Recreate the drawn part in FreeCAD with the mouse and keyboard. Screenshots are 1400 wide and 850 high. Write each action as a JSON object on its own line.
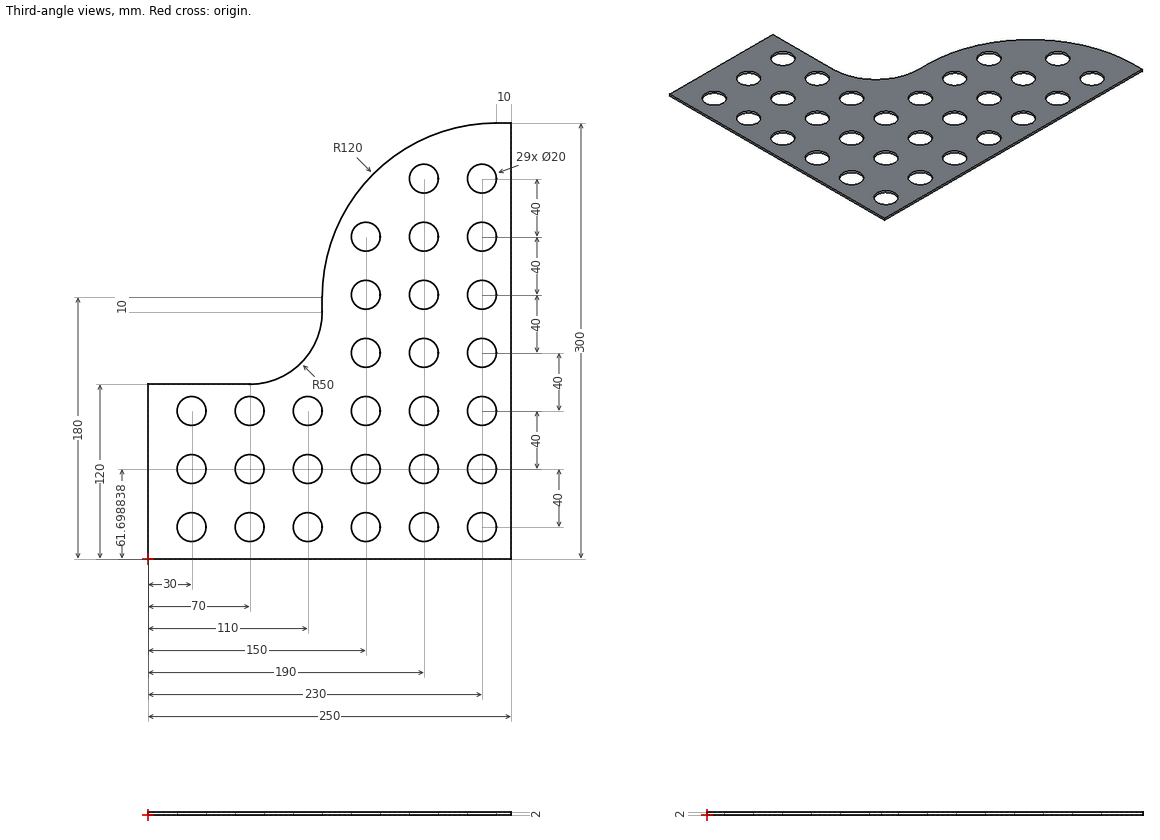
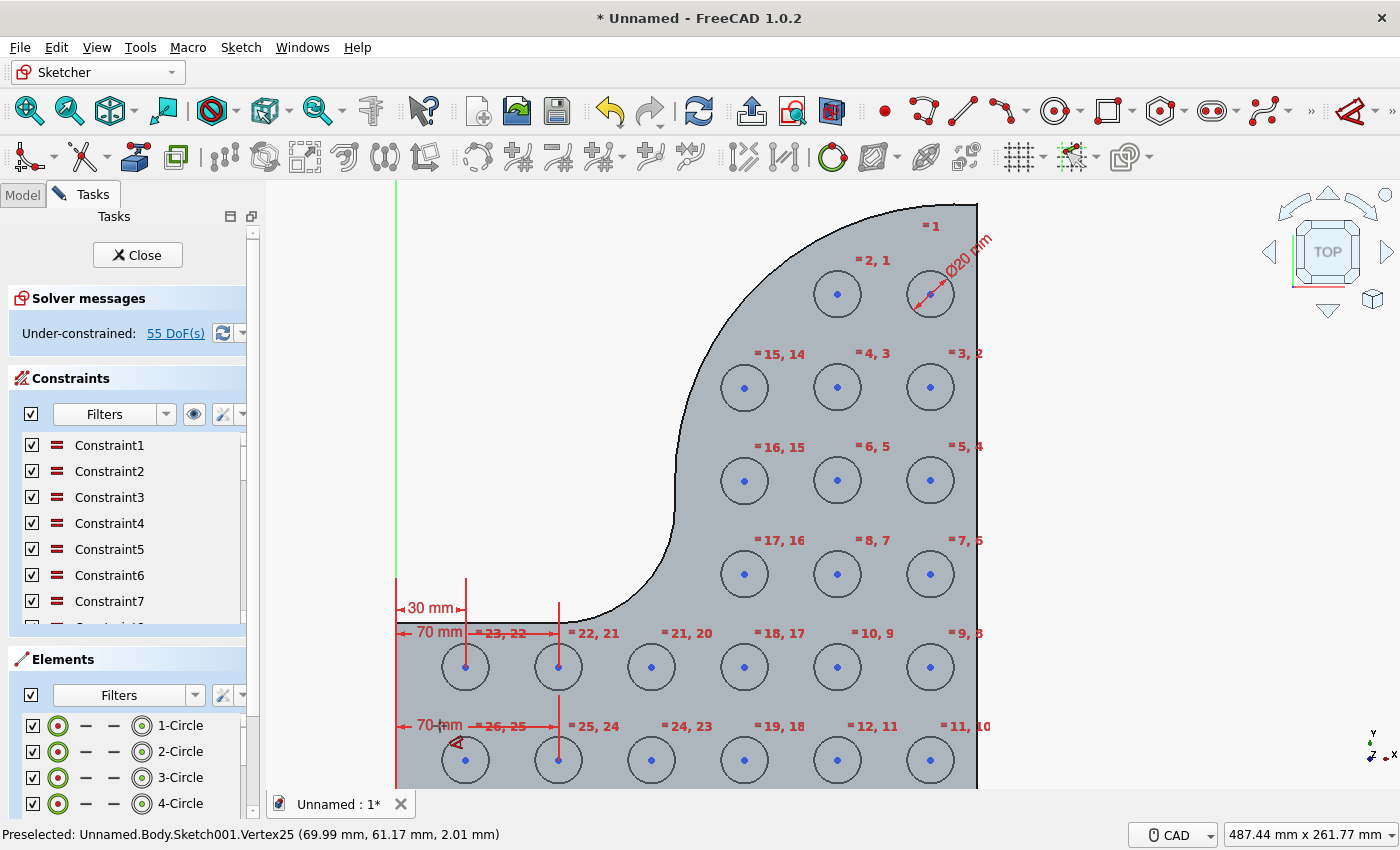
{"action": "left_click", "coordinate": [466, 760]}
{"action": "left_click", "coordinate": [431, 702]}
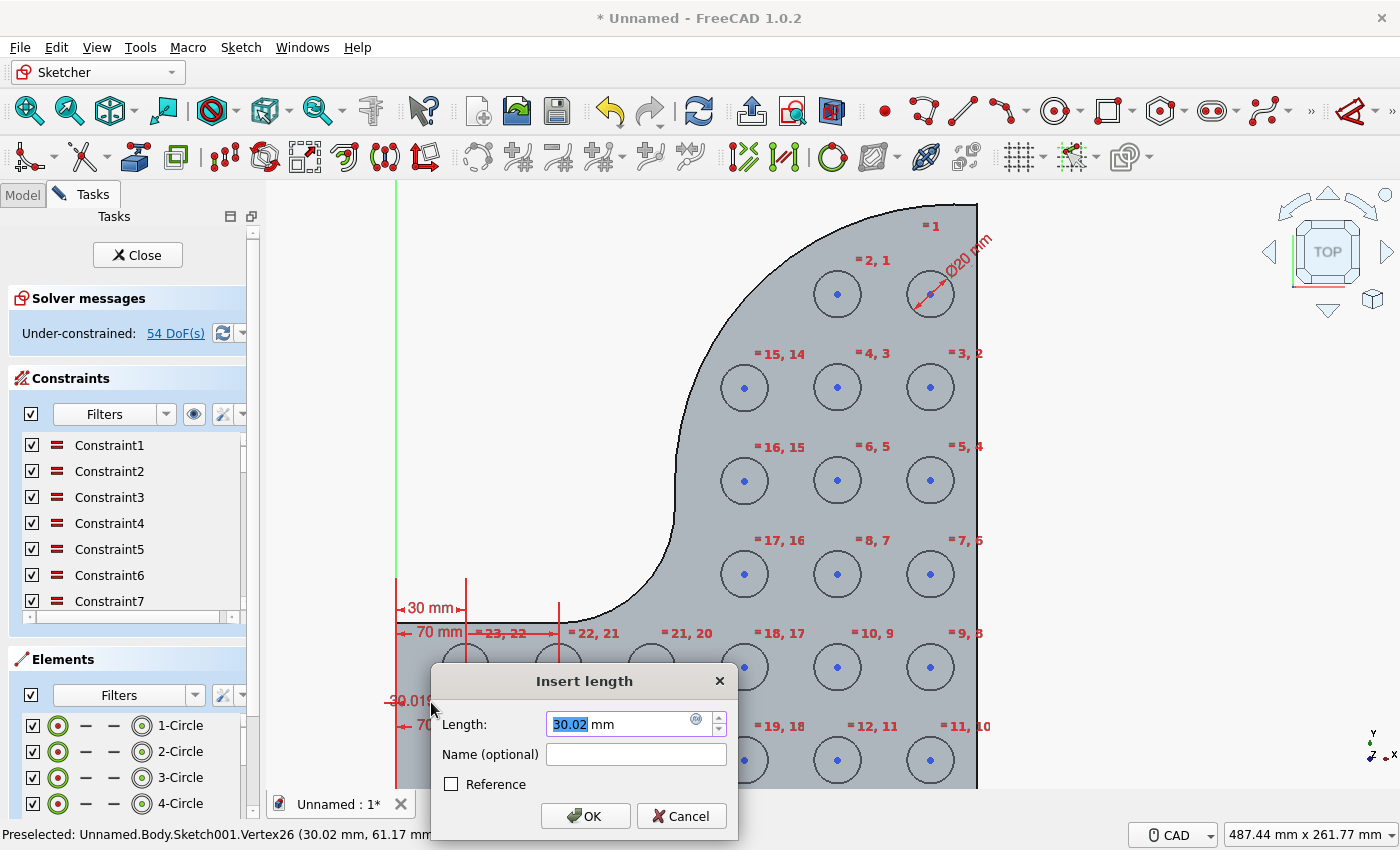
{"action": "type", "text": "30"}
{"action": "key", "text": "Return"}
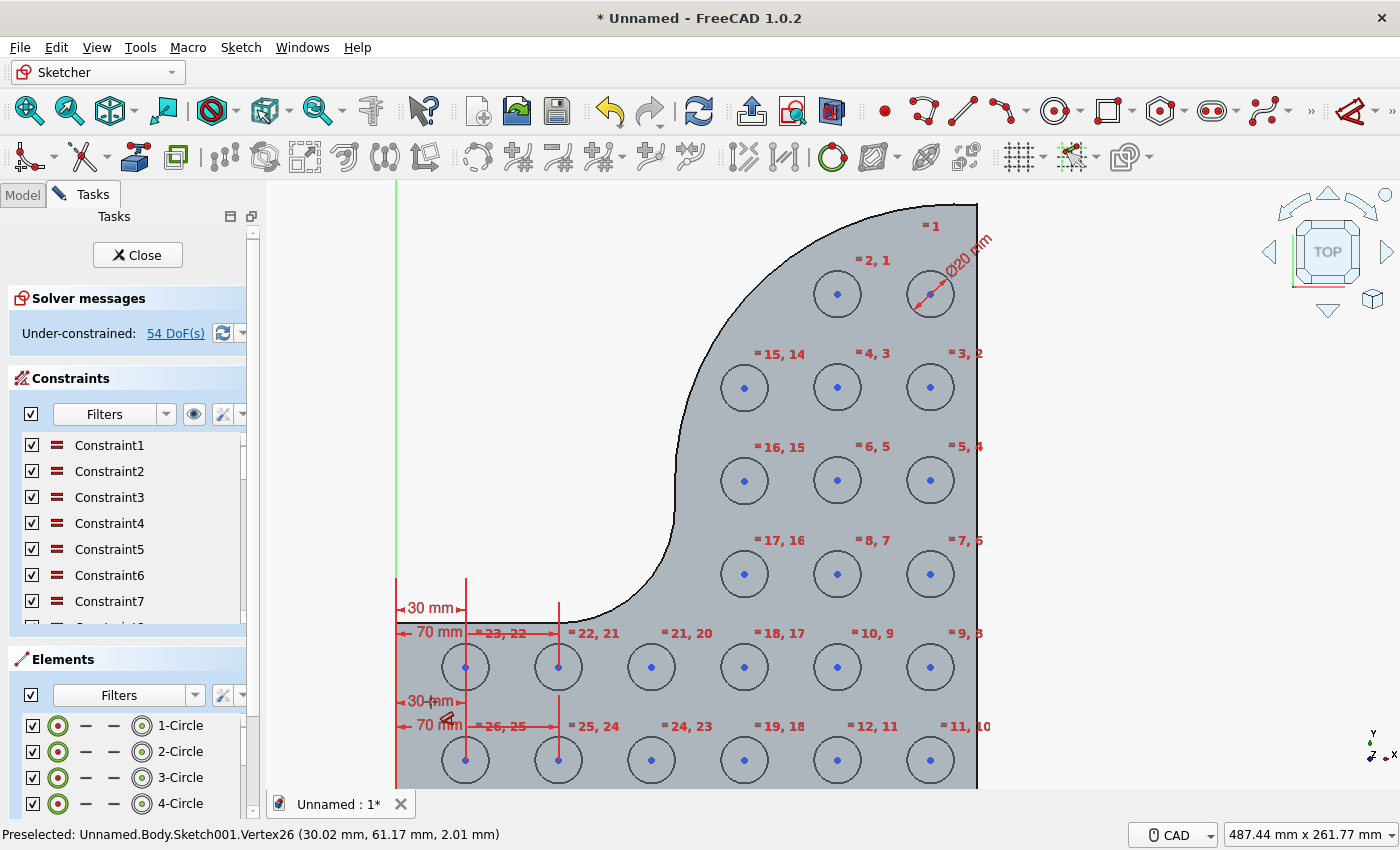
{"action": "scroll", "coordinate": [947, 277], "scroll_direction": "down", "scroll_amount": 2}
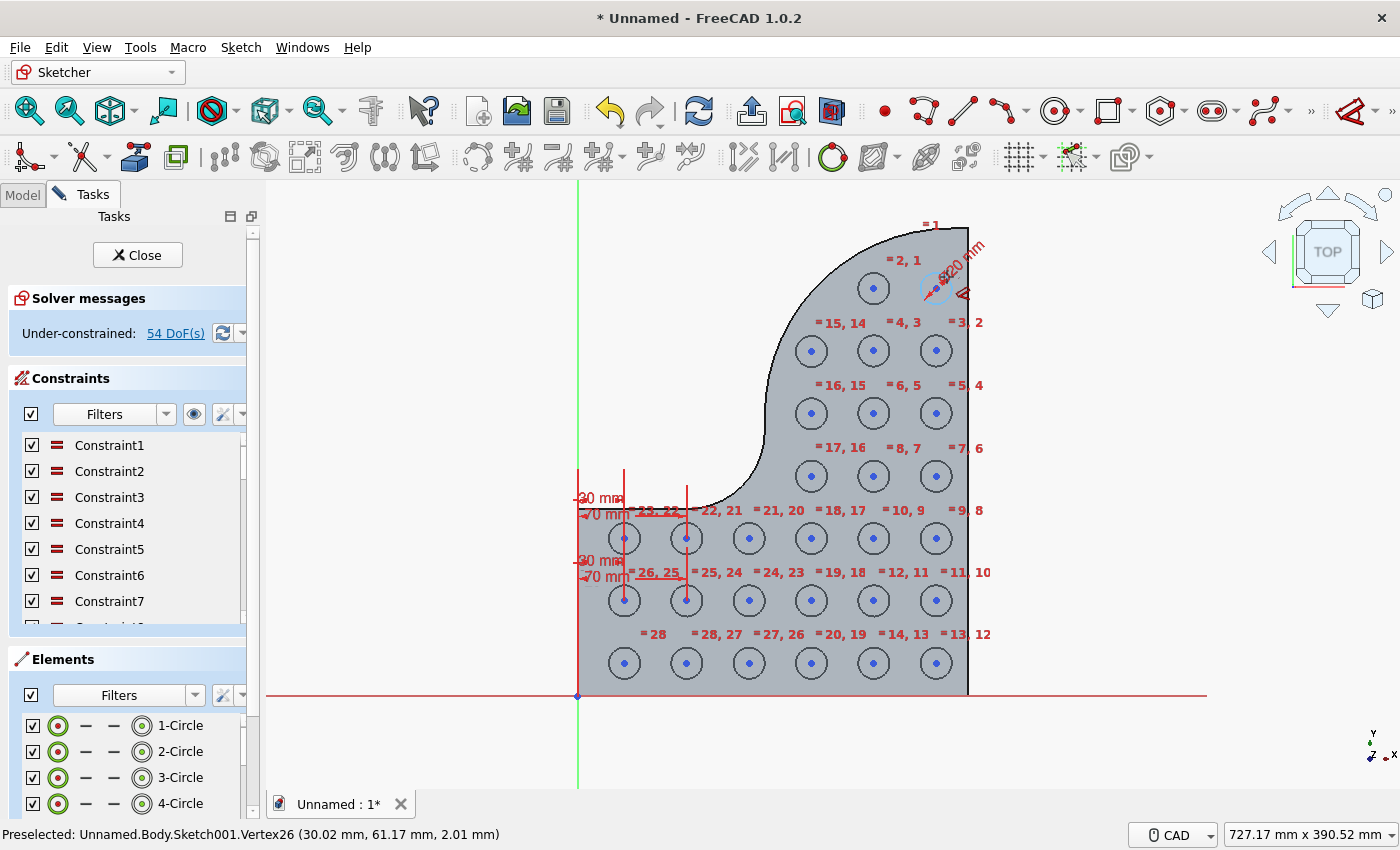
{"action": "left_click", "coordinate": [687, 663]}
{"action": "left_click", "coordinate": [632, 730]}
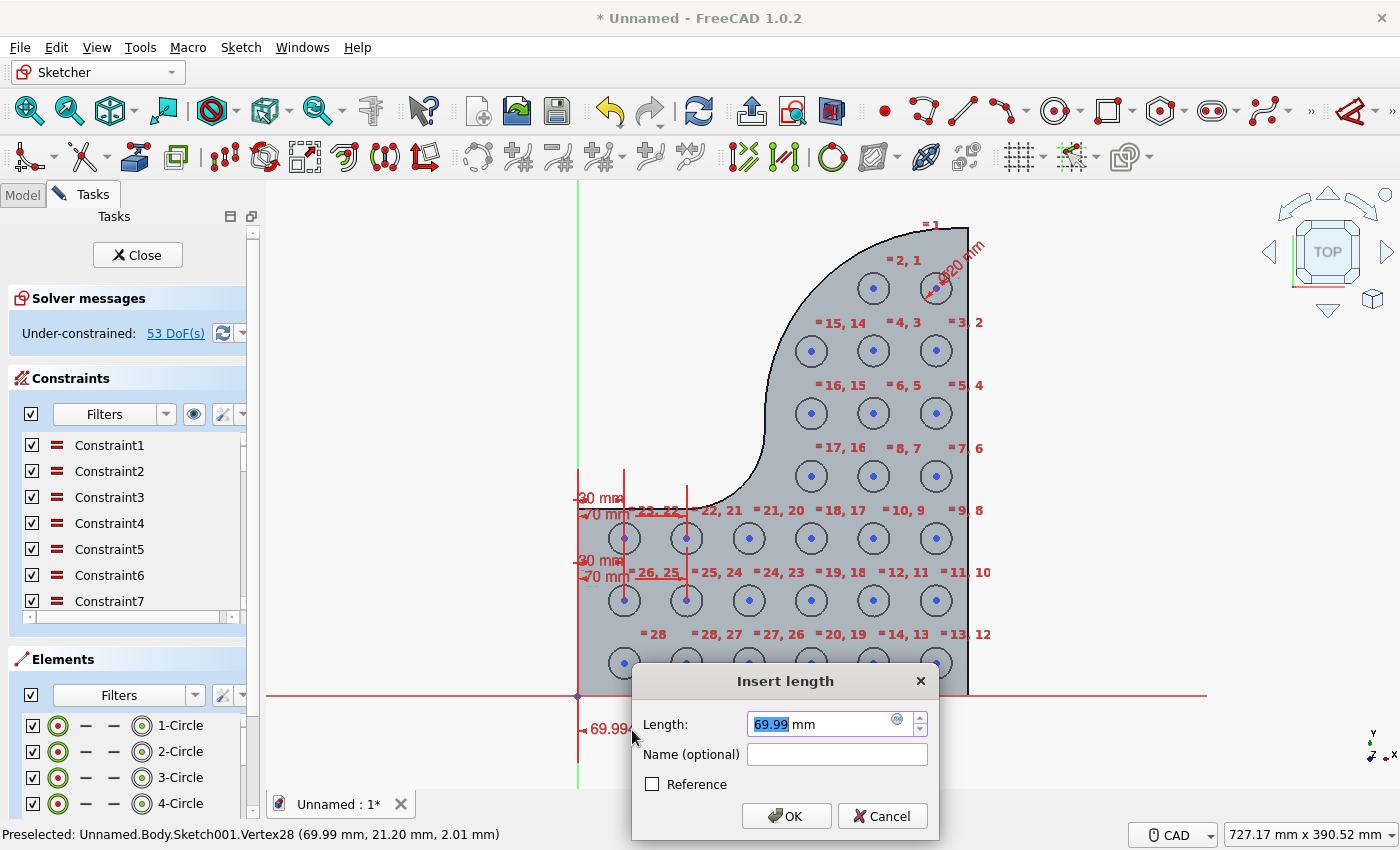
{"action": "type", "text": "70"}
{"action": "key", "text": "Return"}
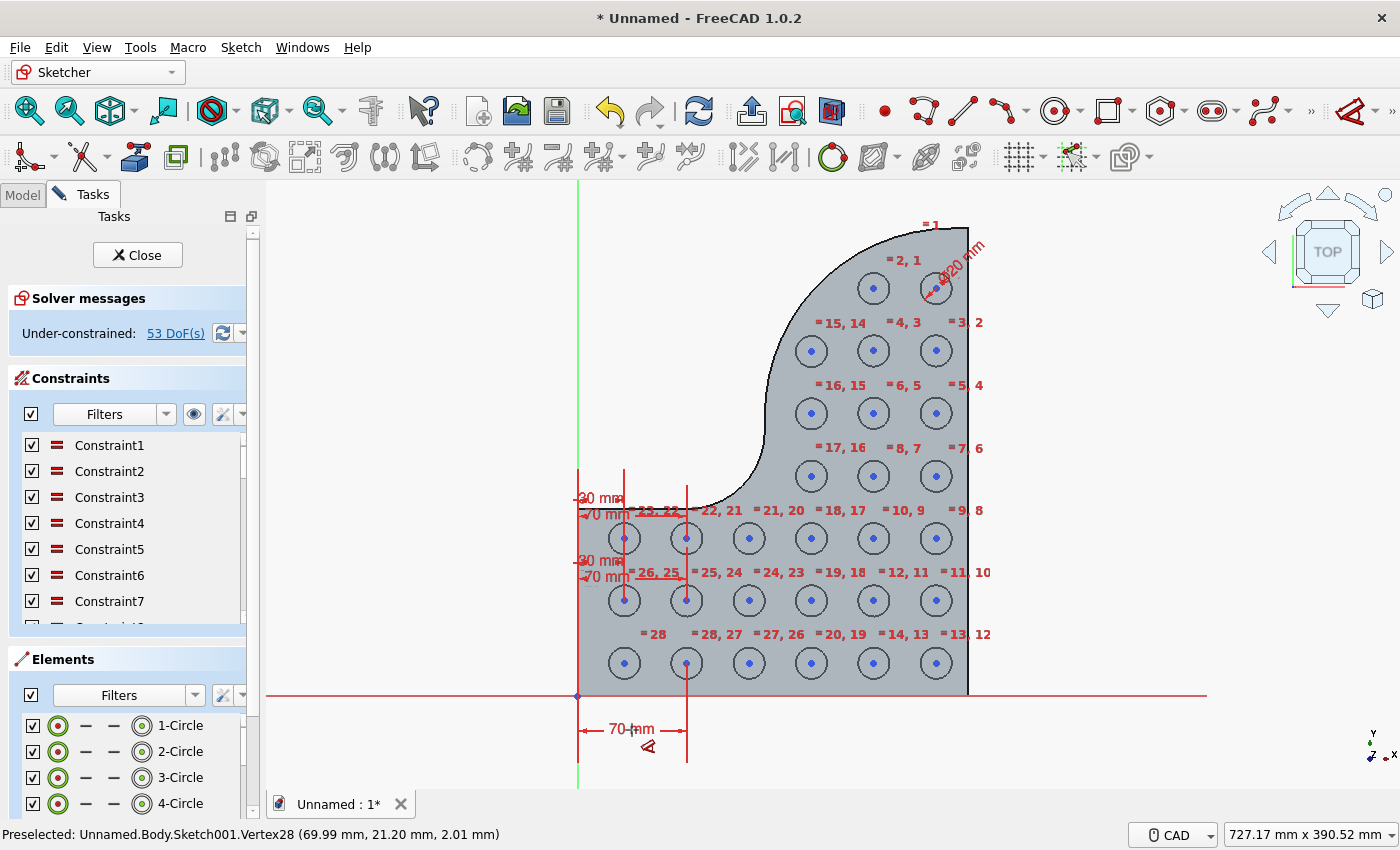
{"action": "left_click", "coordinate": [624, 663]}
{"action": "left_click", "coordinate": [601, 629]}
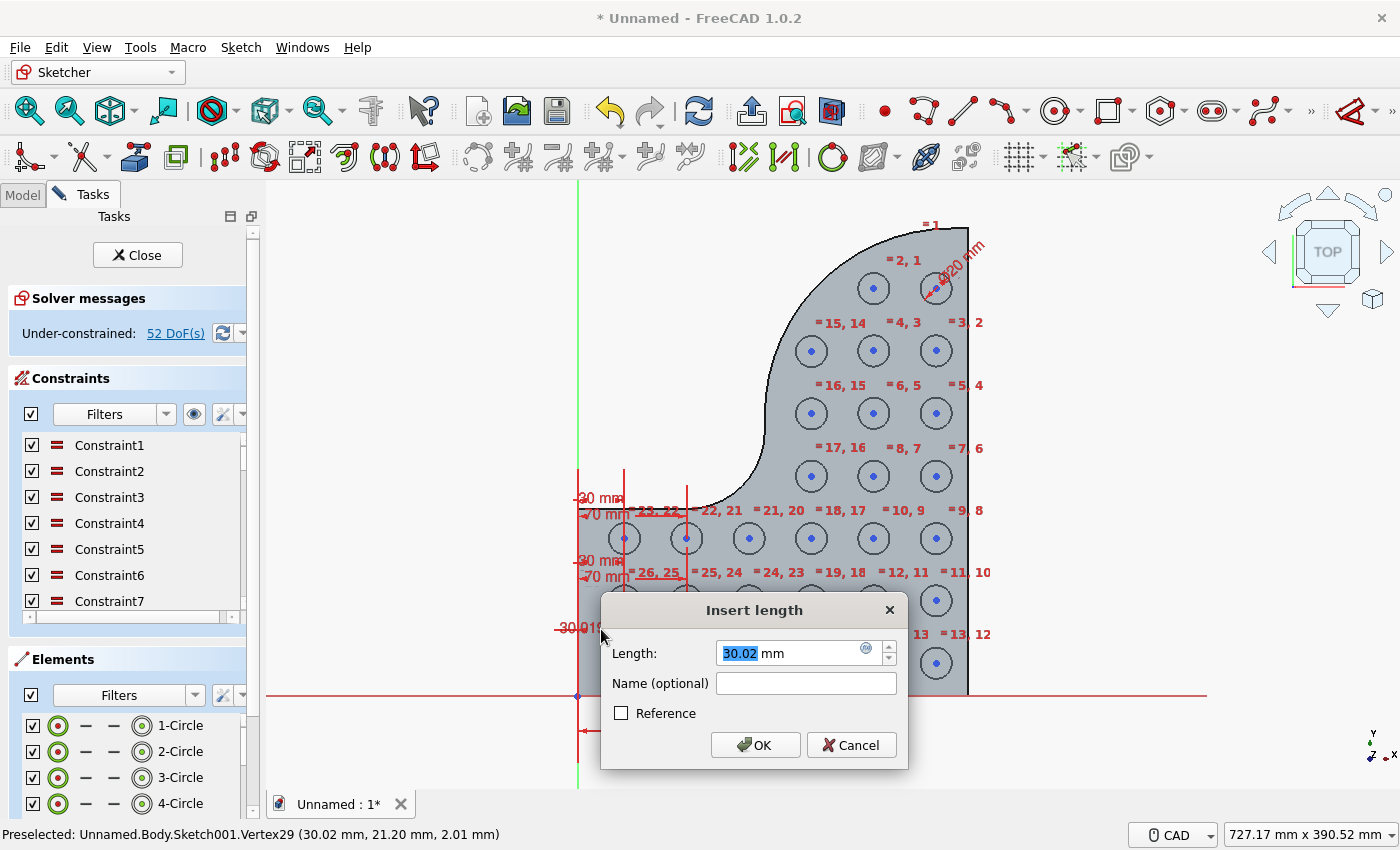
{"action": "type", "text": "30"}
{"action": "key", "text": "Return"}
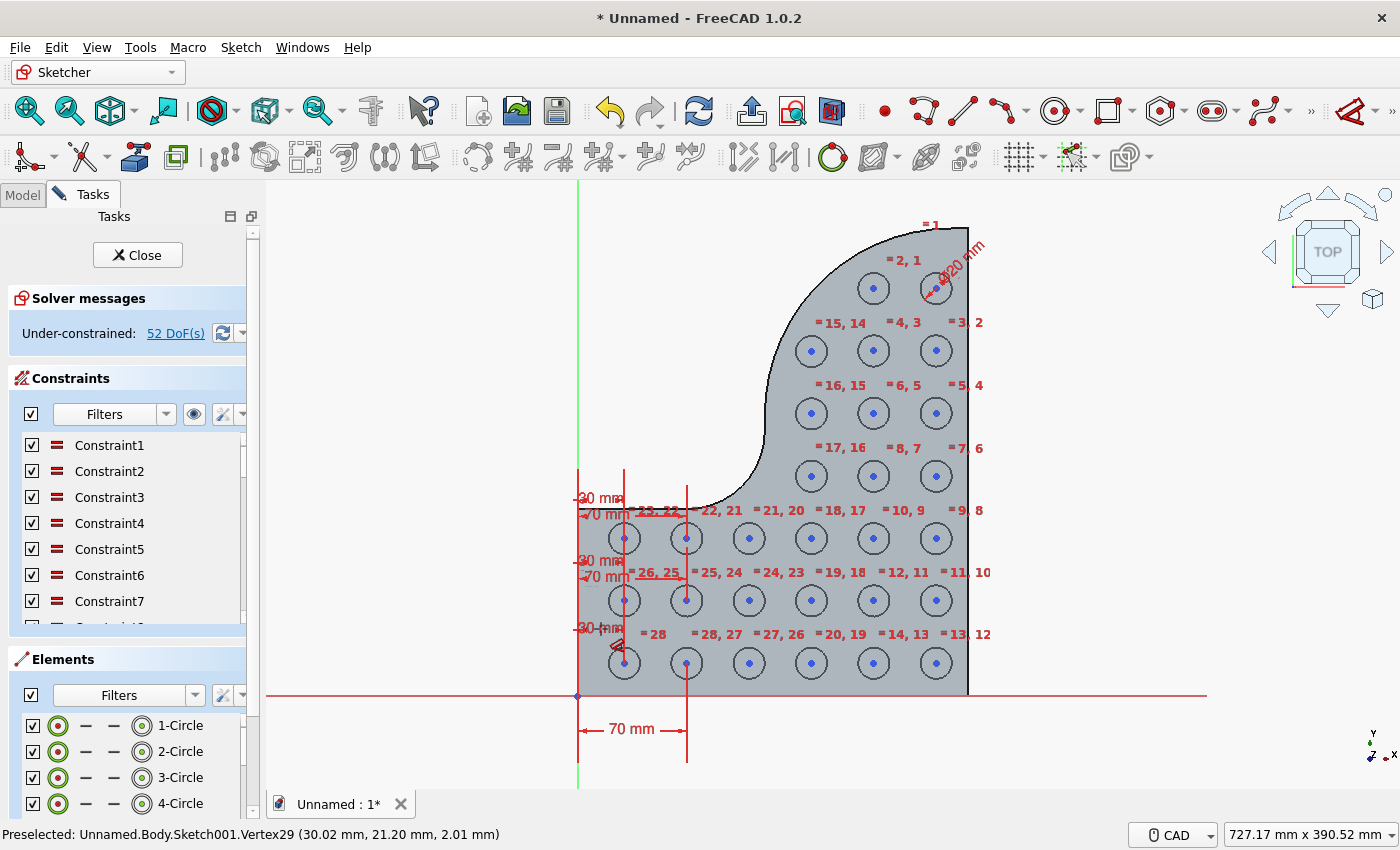
{"action": "left_click", "coordinate": [936, 289]}
{"action": "left_click", "coordinate": [757, 730]}